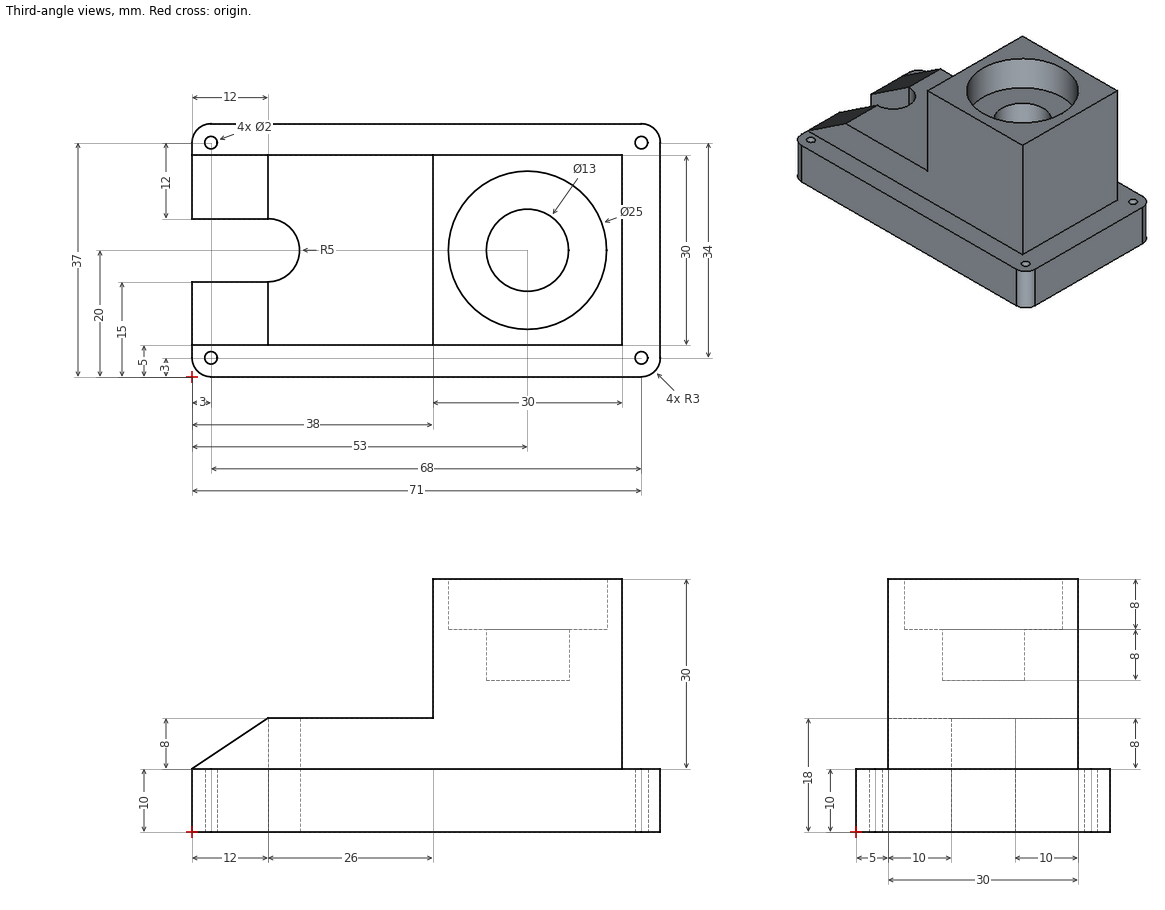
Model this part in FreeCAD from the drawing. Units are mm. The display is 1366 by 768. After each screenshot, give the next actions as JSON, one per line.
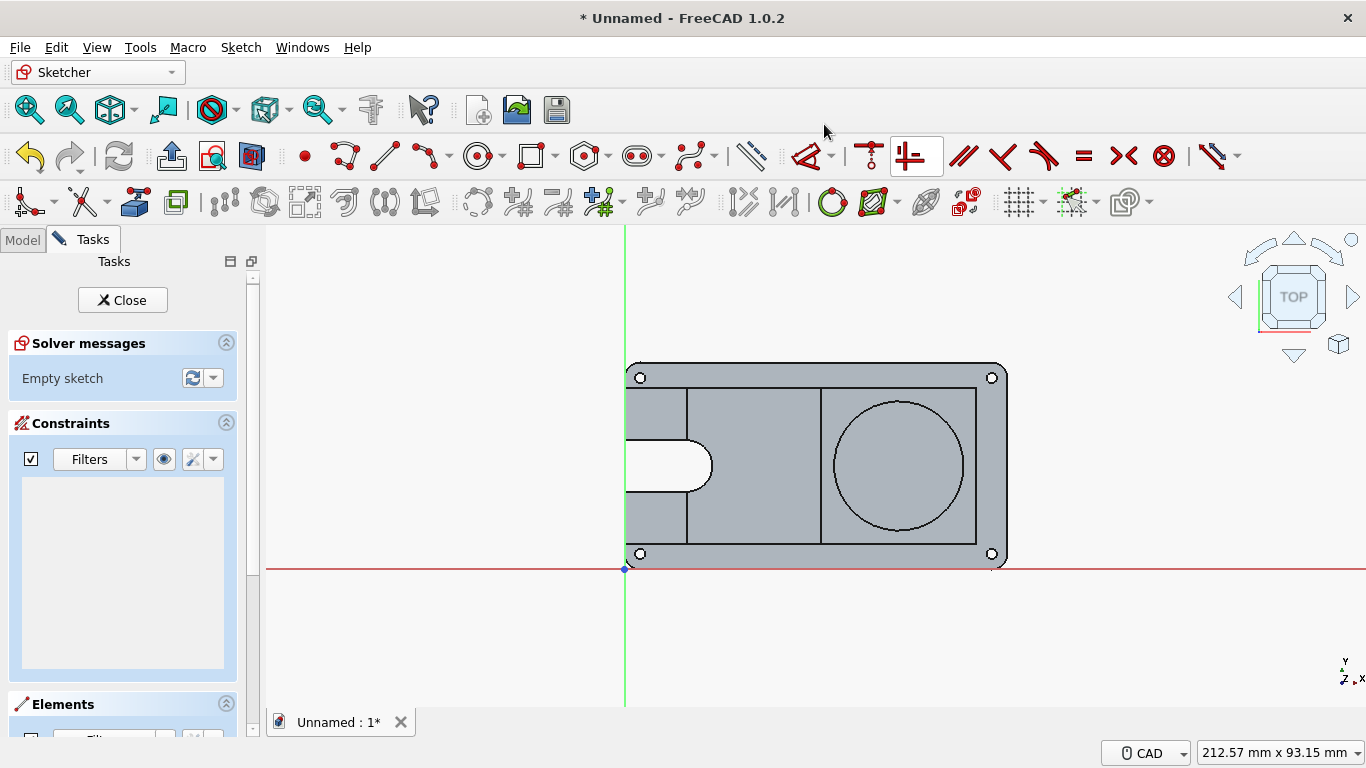
{"action": "left_click", "coordinate": [252, 156]}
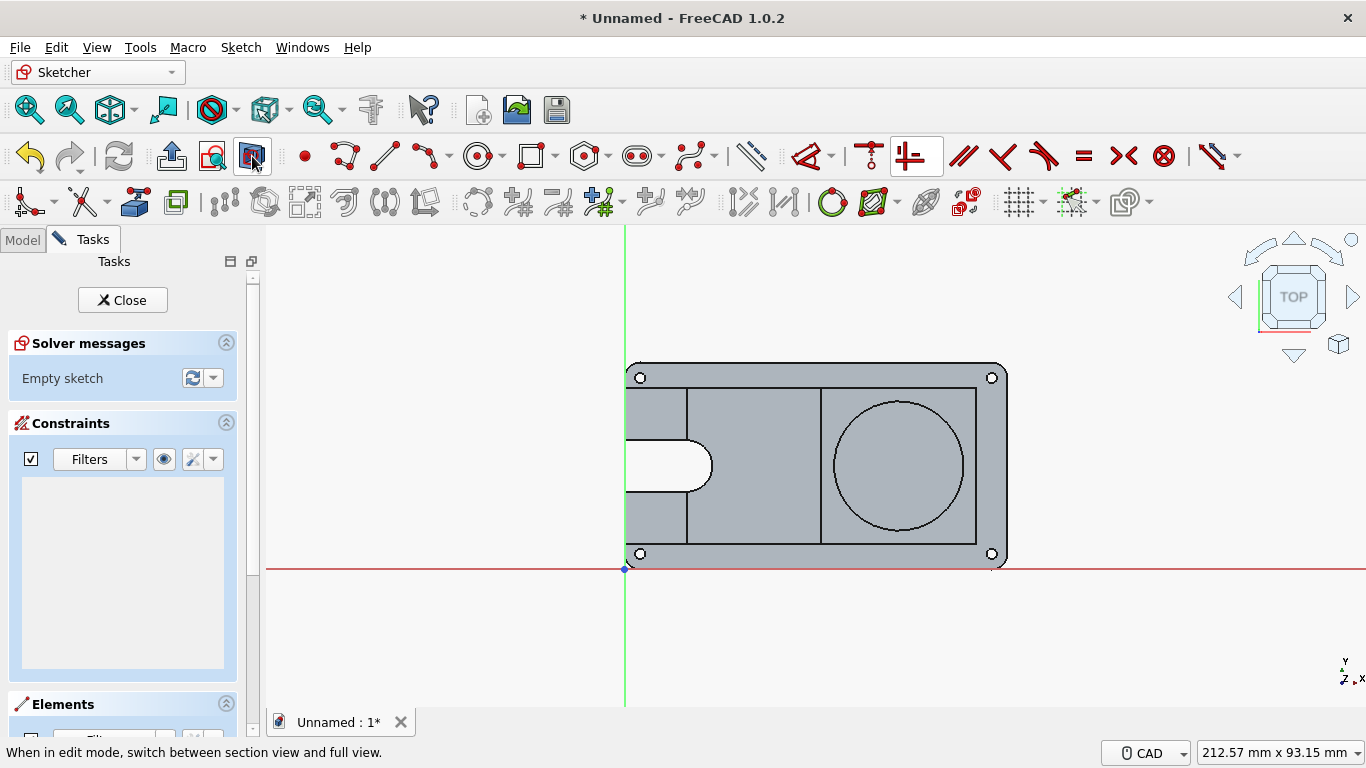
{"action": "scroll", "coordinate": [948, 466], "scroll_direction": "up", "scroll_amount": 7}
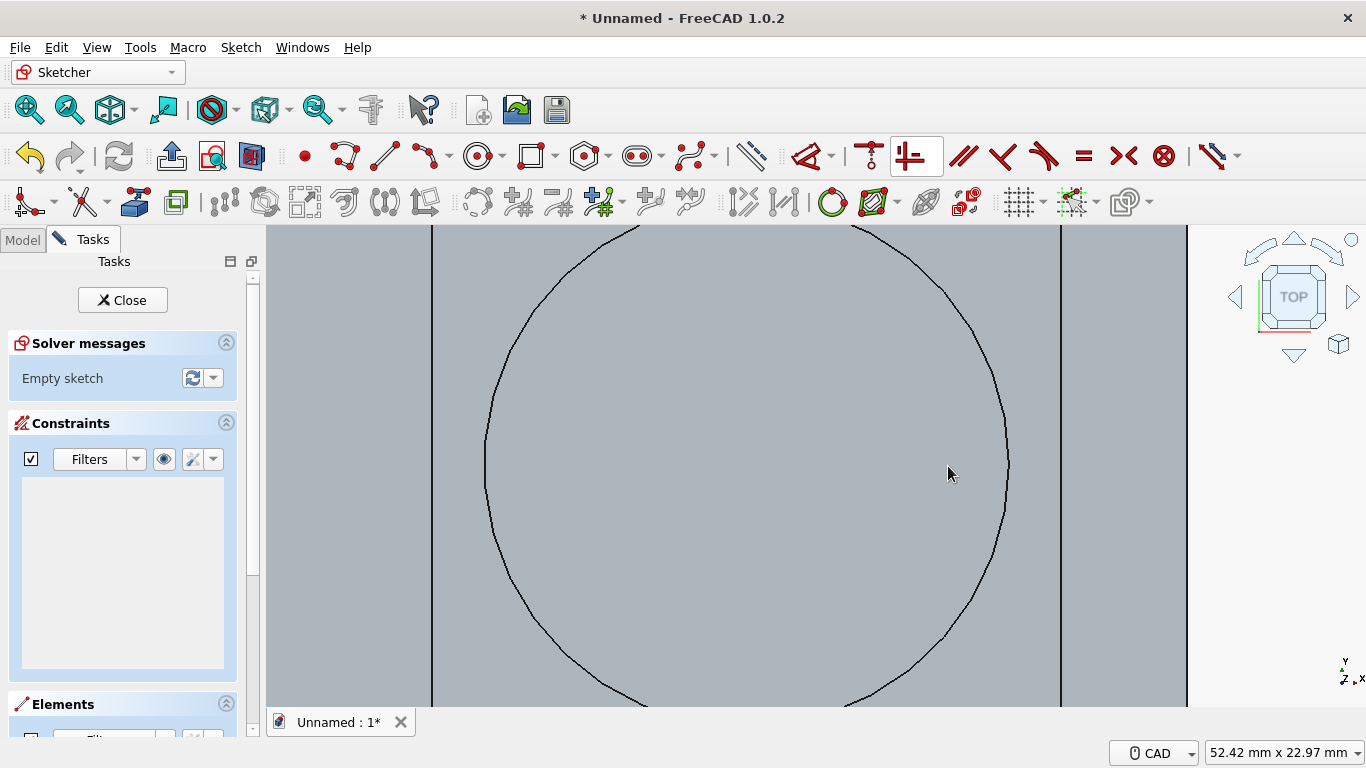
{"action": "left_click", "coordinate": [478, 156]}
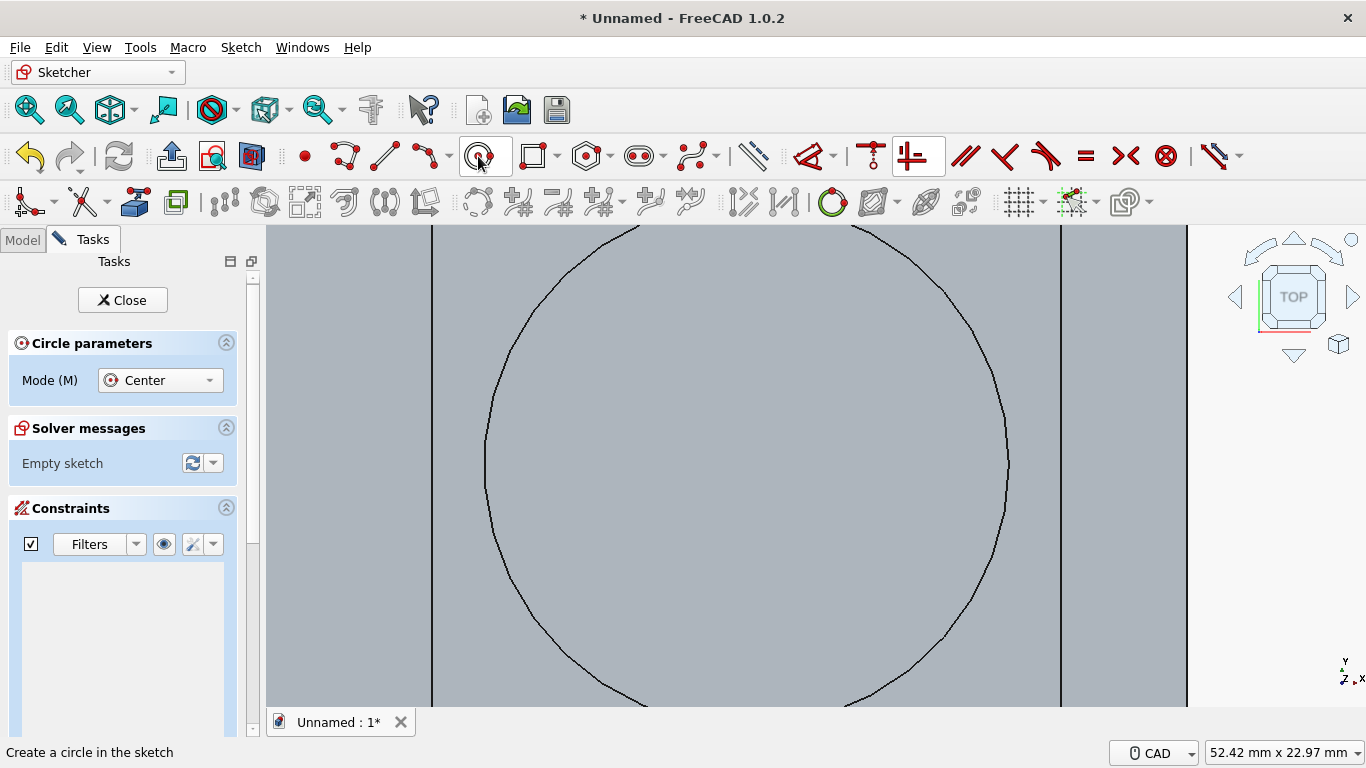
{"action": "left_click", "coordinate": [747, 464]}
{"action": "left_click", "coordinate": [843, 368]}
{"action": "key", "text": "Escape"}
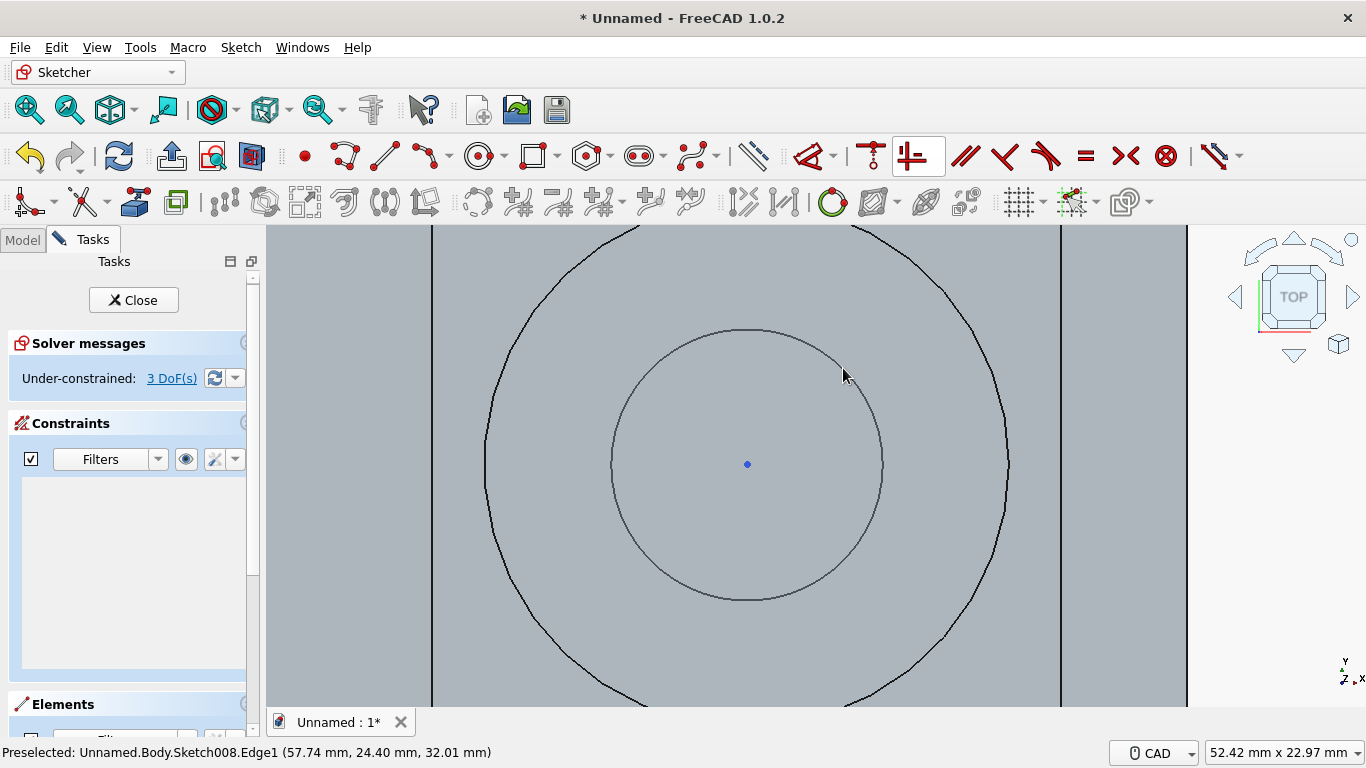
{"action": "left_click", "coordinate": [808, 156]}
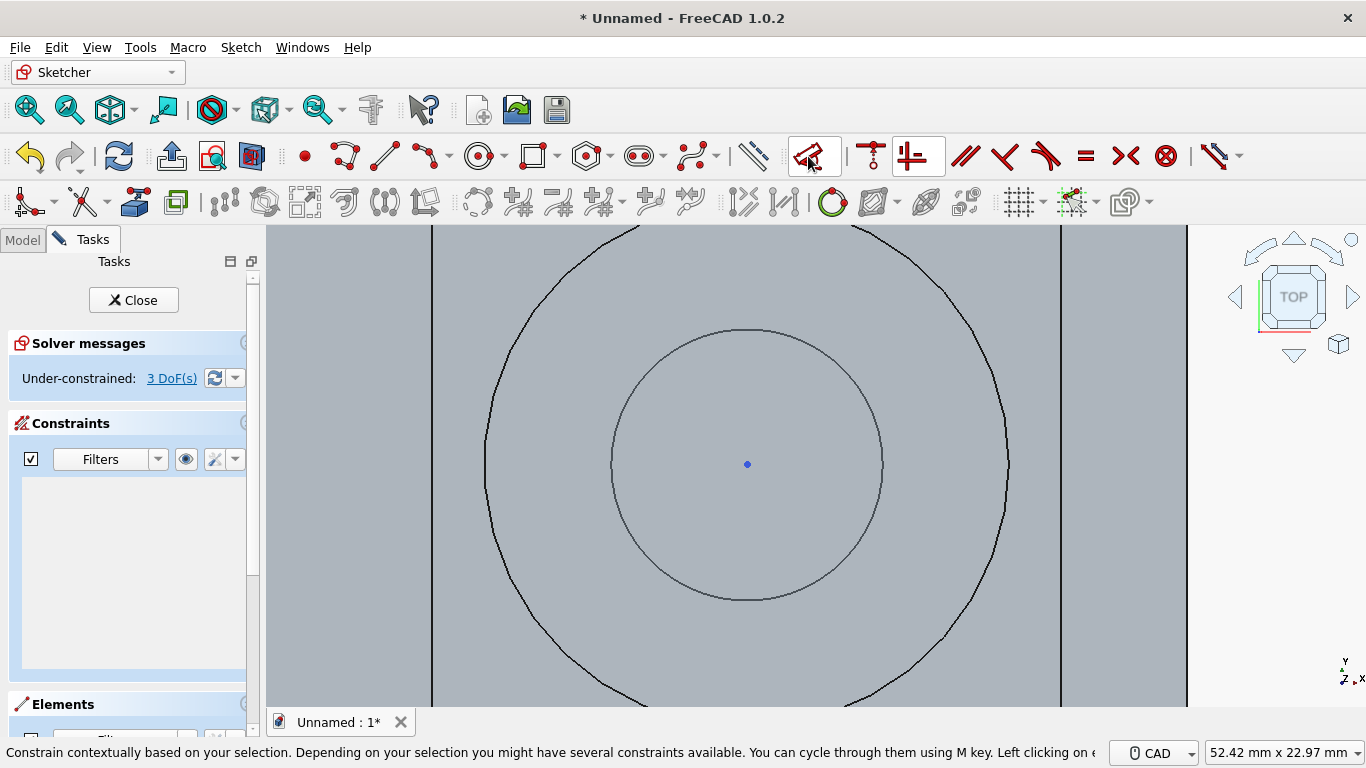
{"action": "left_click", "coordinate": [843, 369]}
{"action": "left_click", "coordinate": [866, 346]}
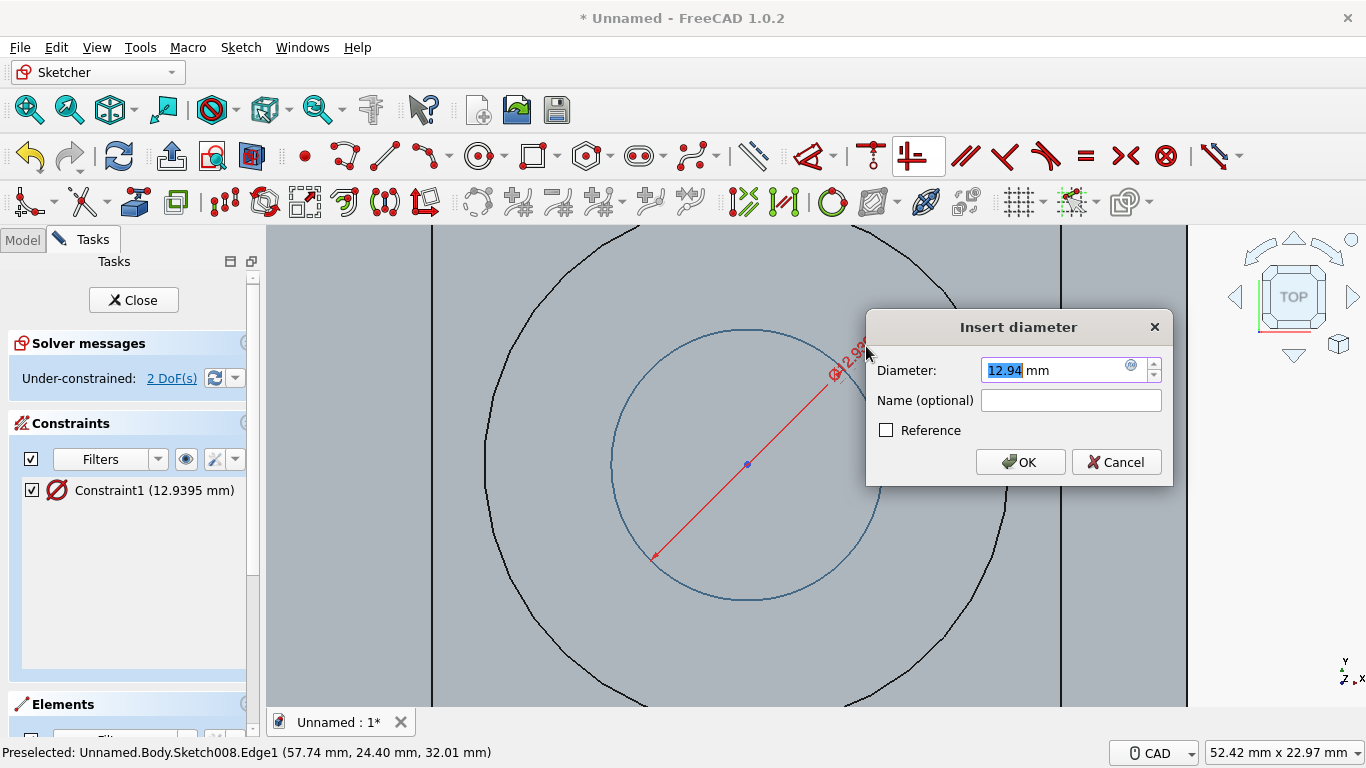
{"action": "type", "text": "13"}
{"action": "key", "text": "Return"}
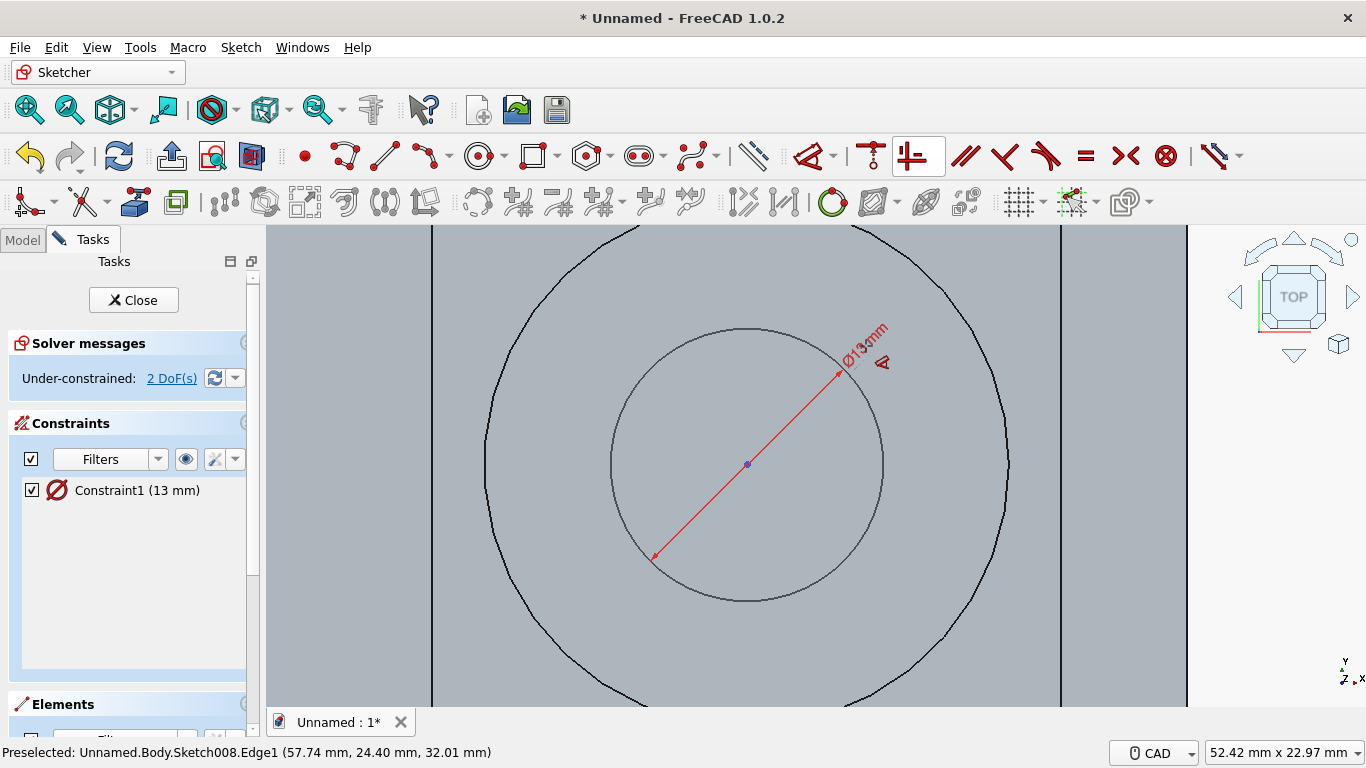
{"action": "left_click", "coordinate": [747, 465]}
{"action": "left_click", "coordinate": [520, 431]}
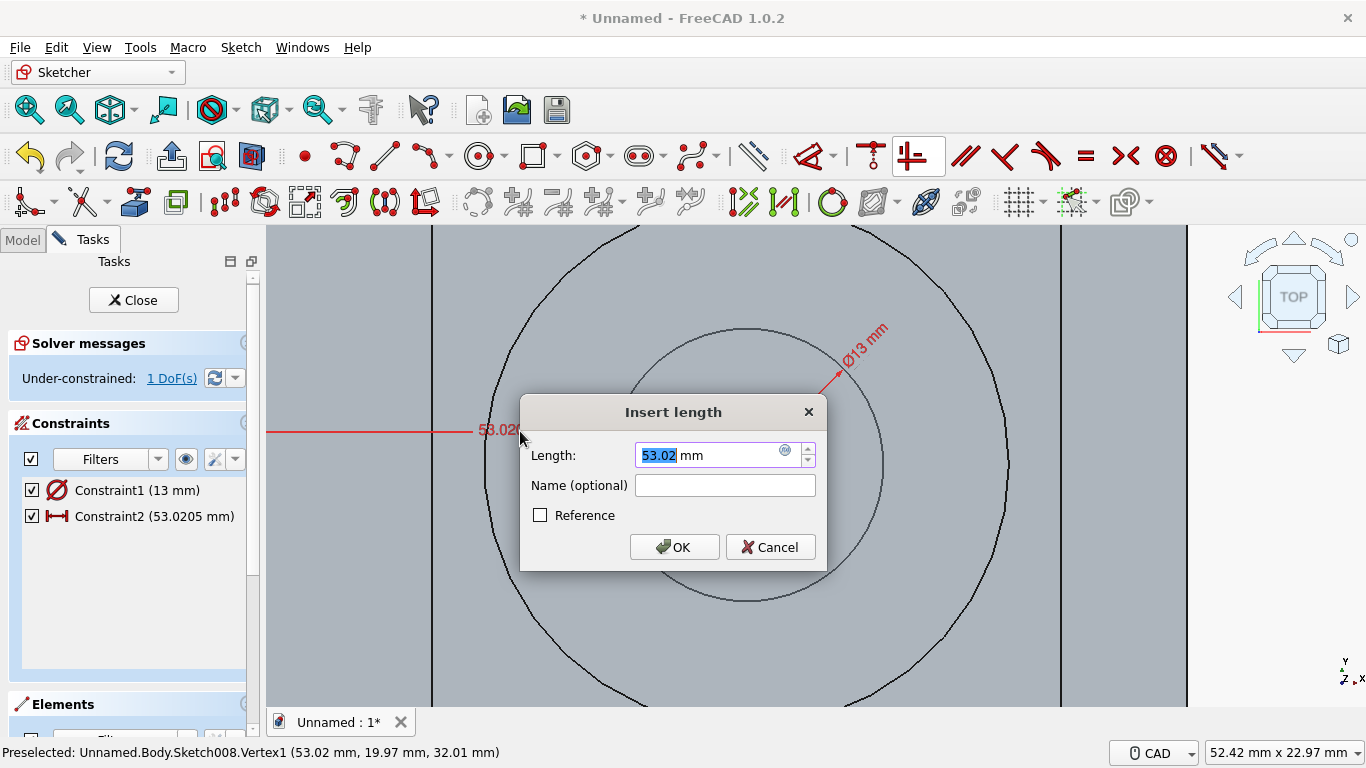
{"action": "type", "text": "53"}
{"action": "key", "text": "Return"}